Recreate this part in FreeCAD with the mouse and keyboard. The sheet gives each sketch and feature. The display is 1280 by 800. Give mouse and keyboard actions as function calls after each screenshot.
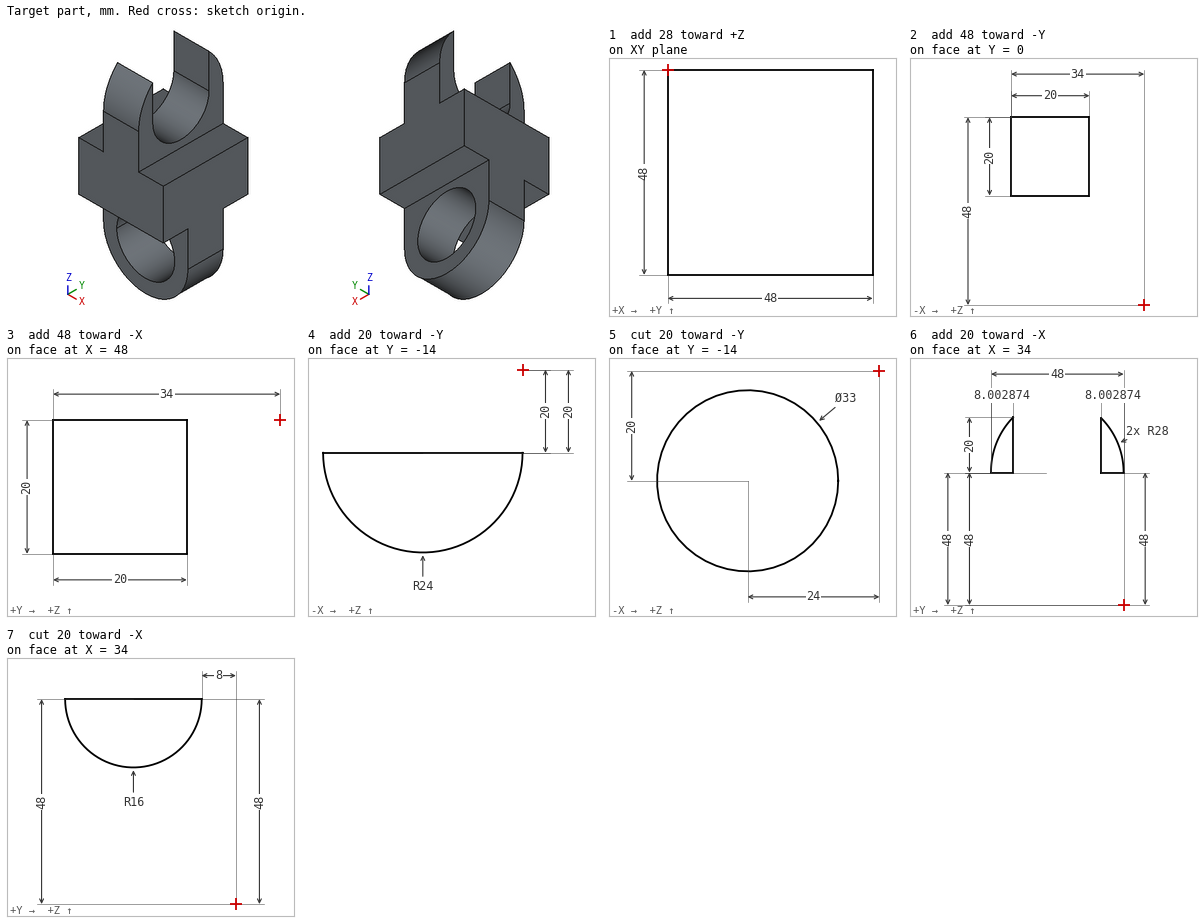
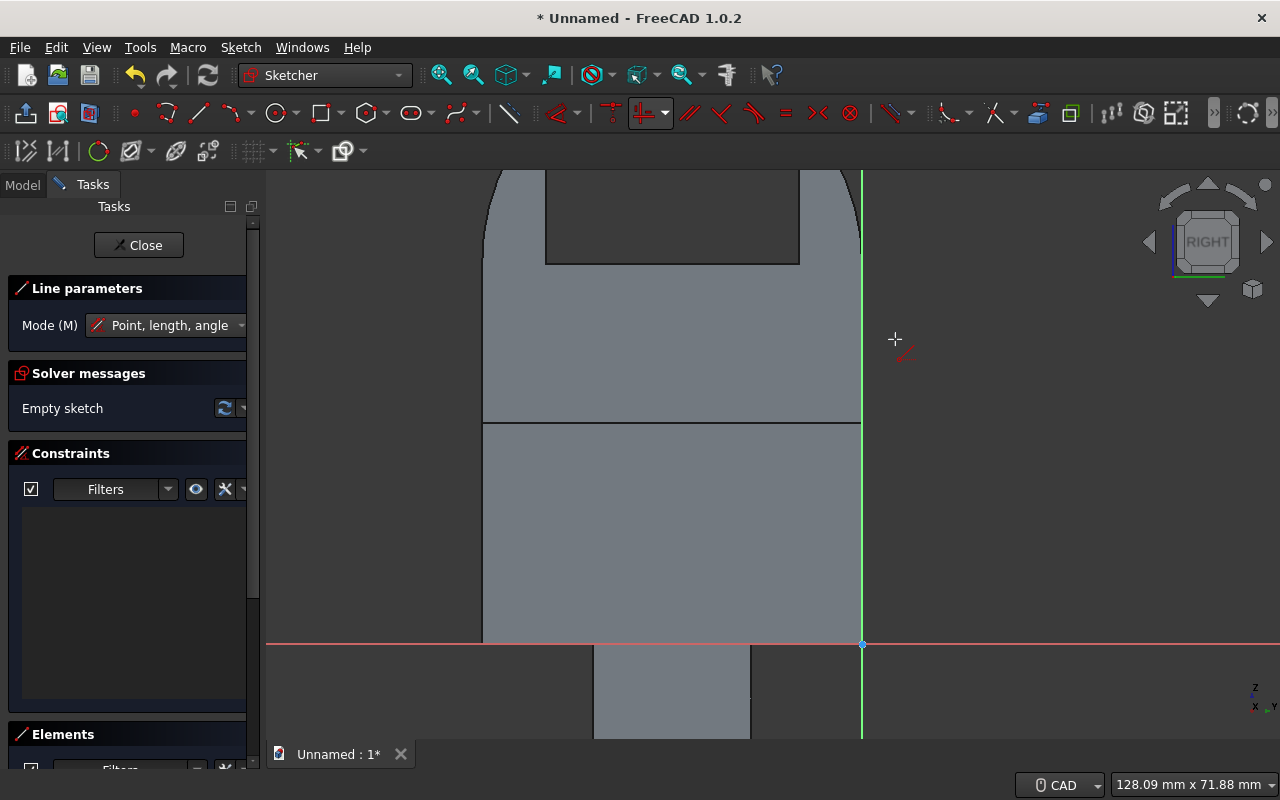
click(799, 264)
click(546, 264)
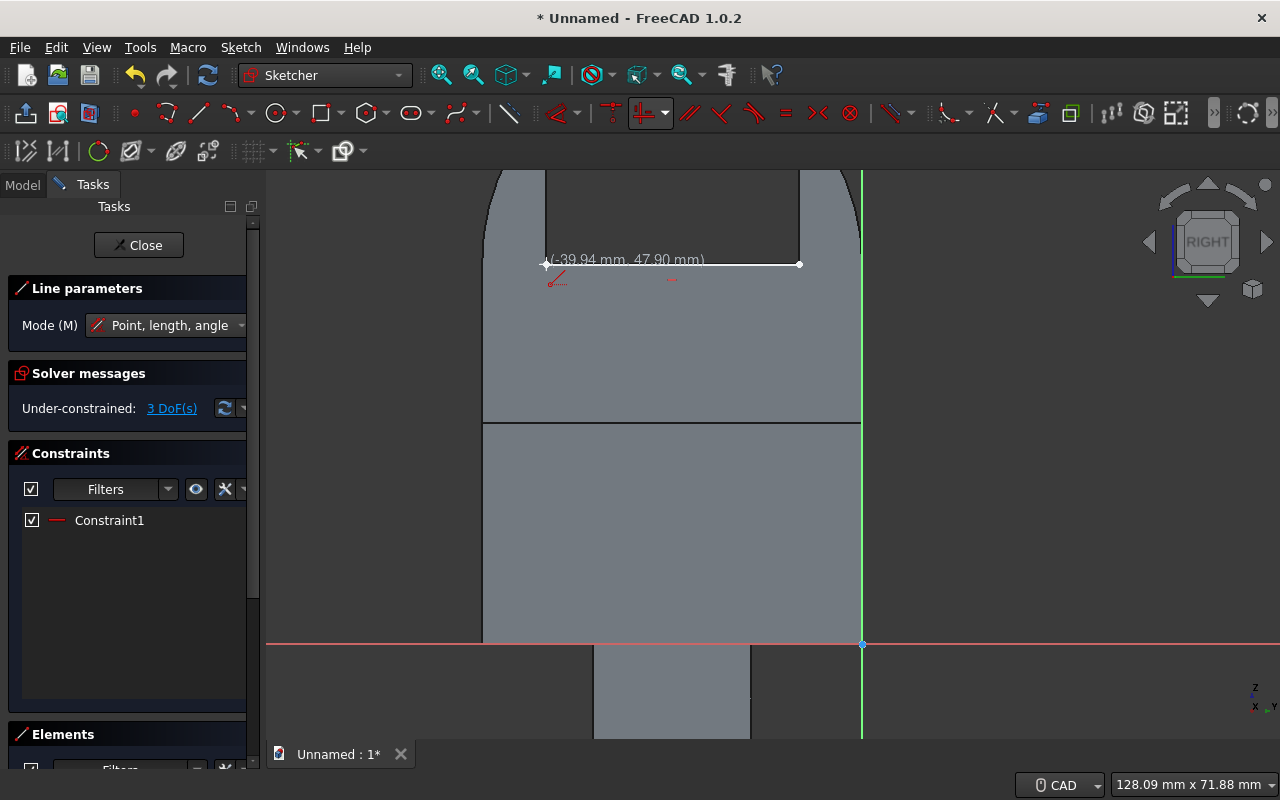
key(g)
key(3)
key(a)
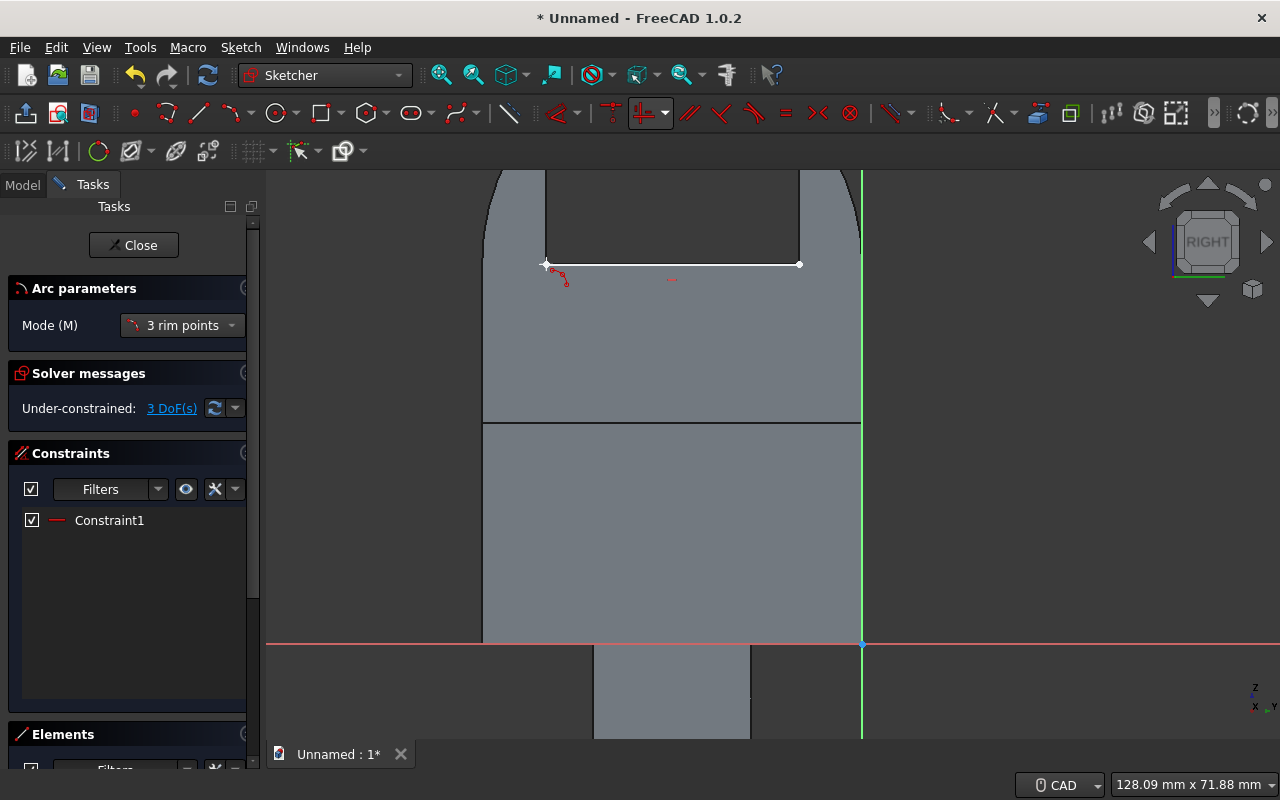
click(546, 265)
click(799, 265)
click(672, 391)
key(Escape)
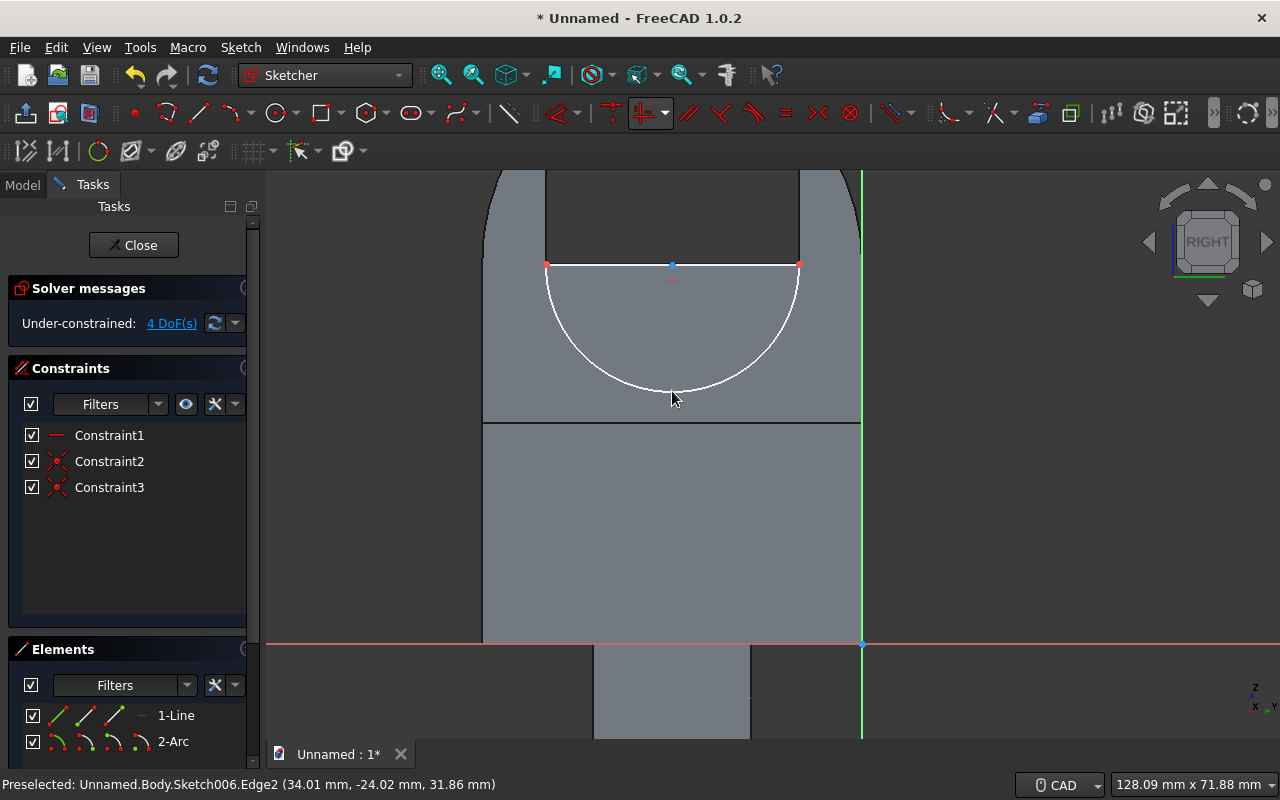
key(d)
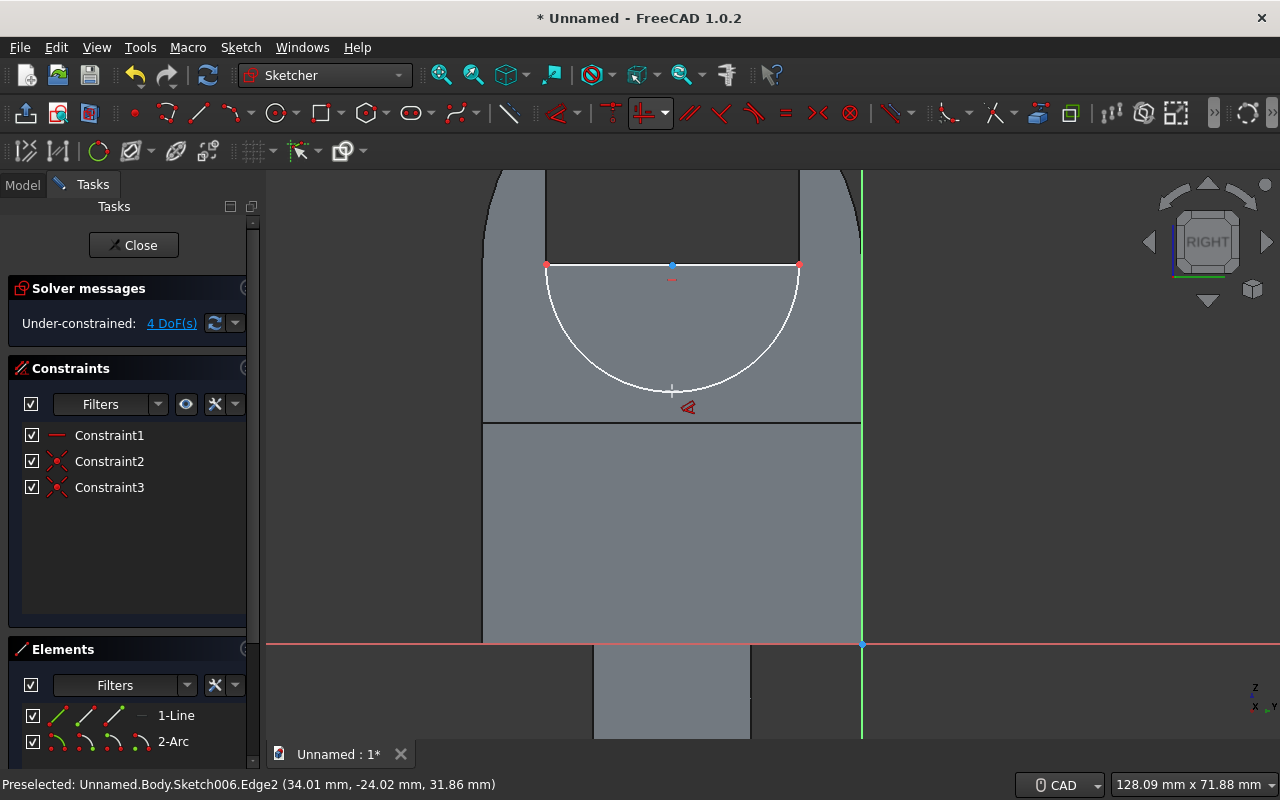
click(598, 368)
click(579, 394)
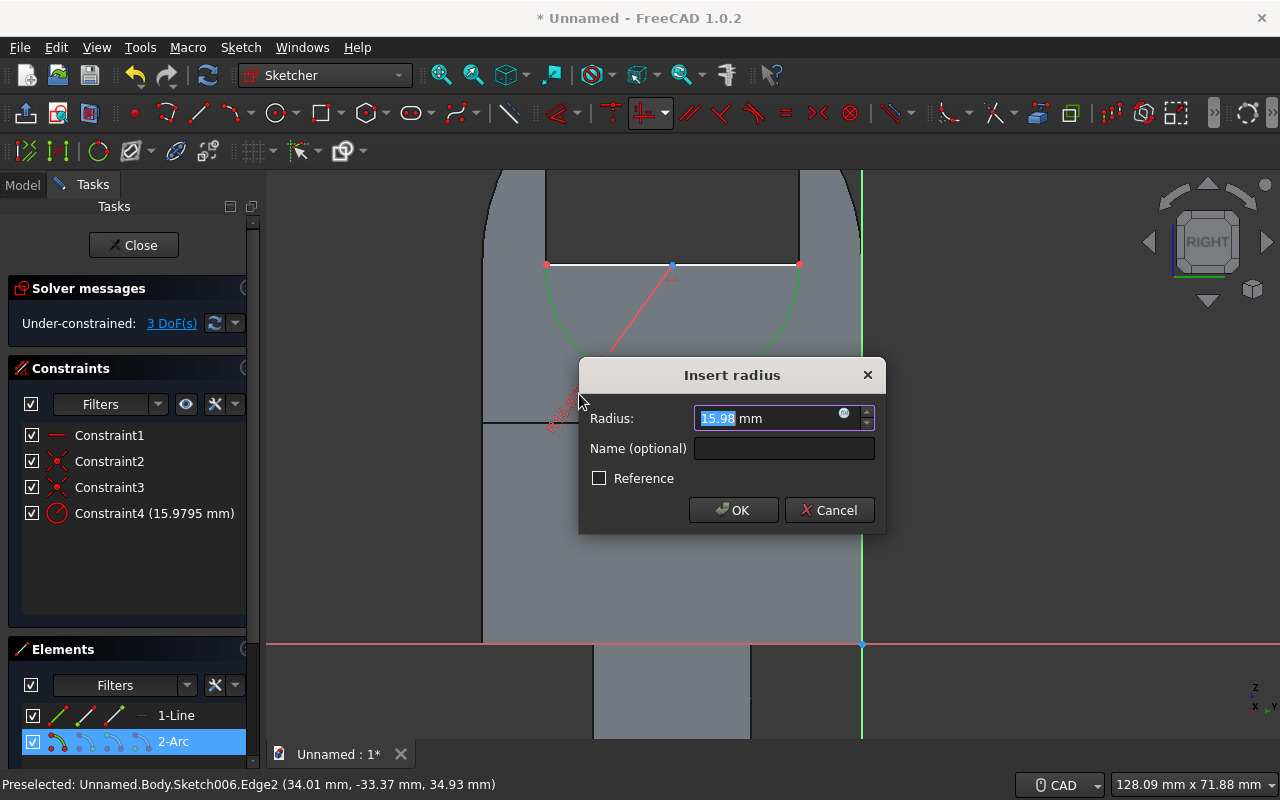
text(16)
key(Return)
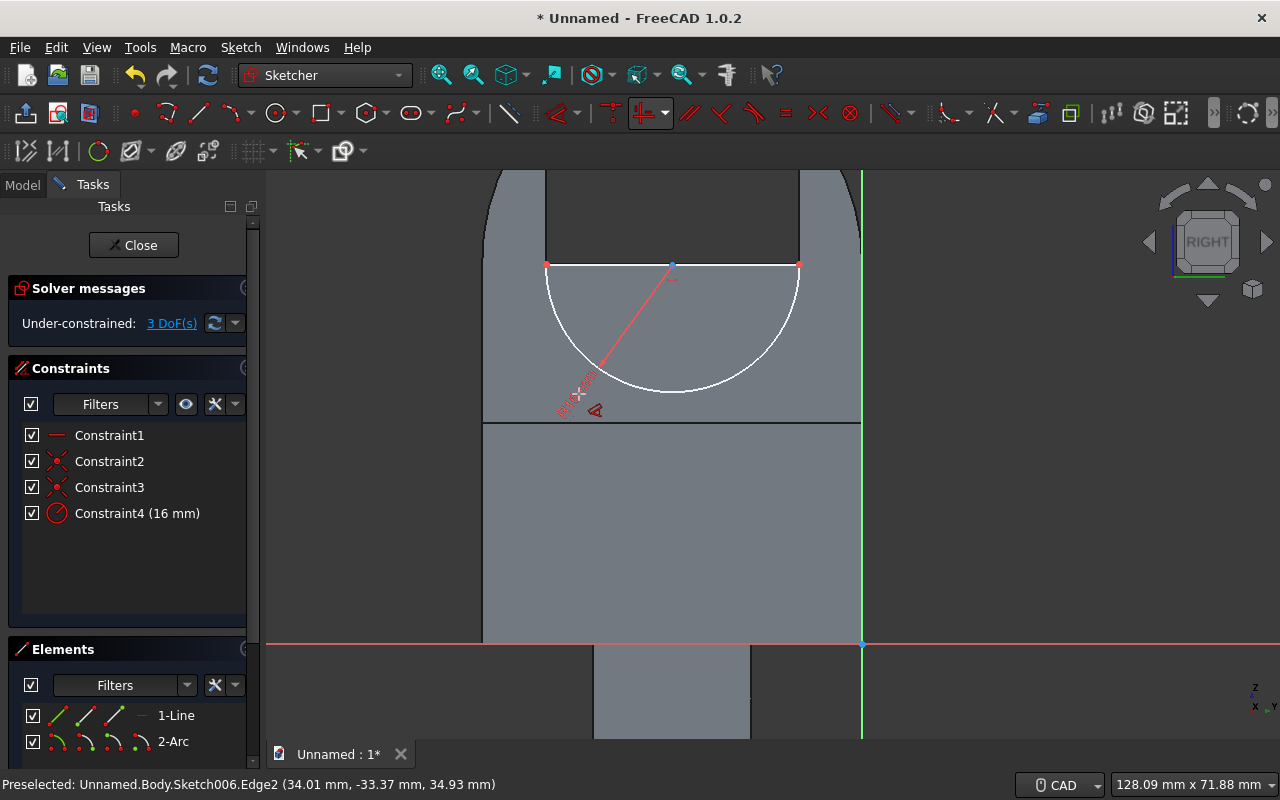
click(799, 265)
click(831, 678)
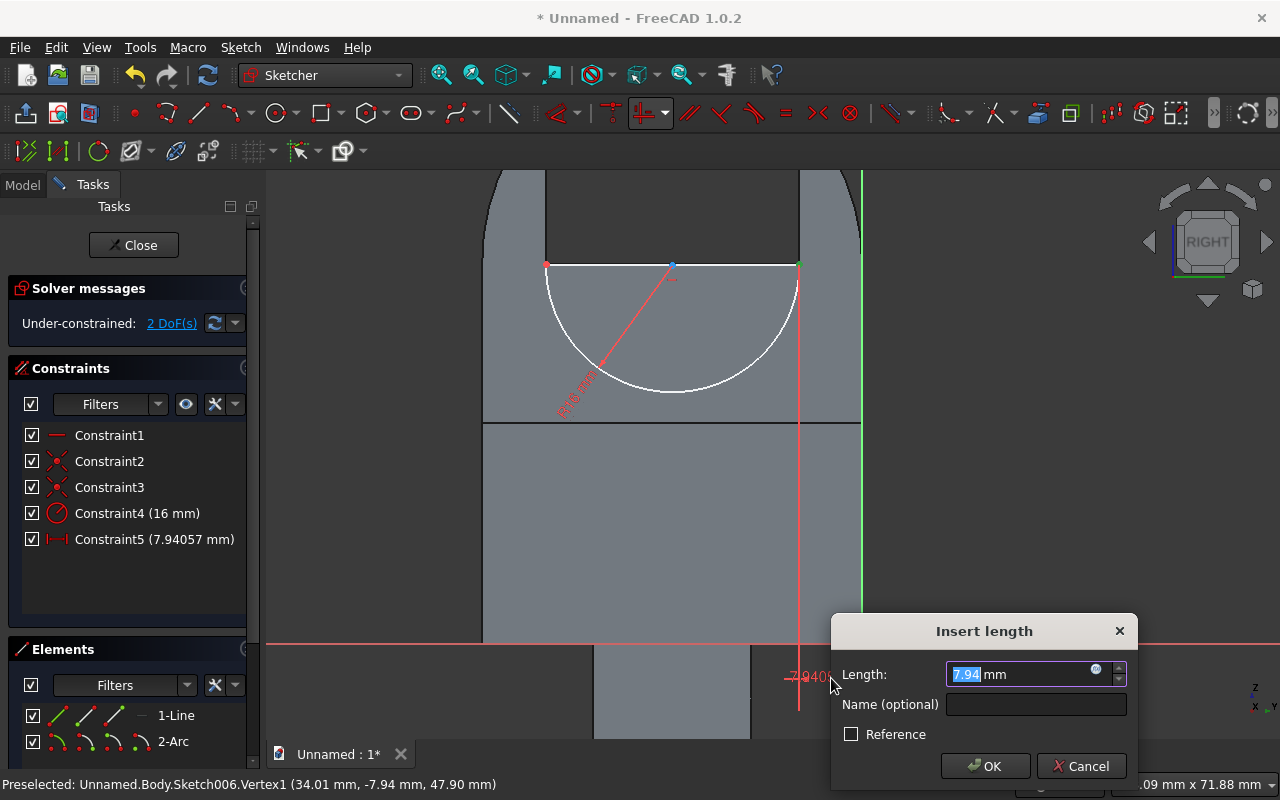
text(8)
key(Return)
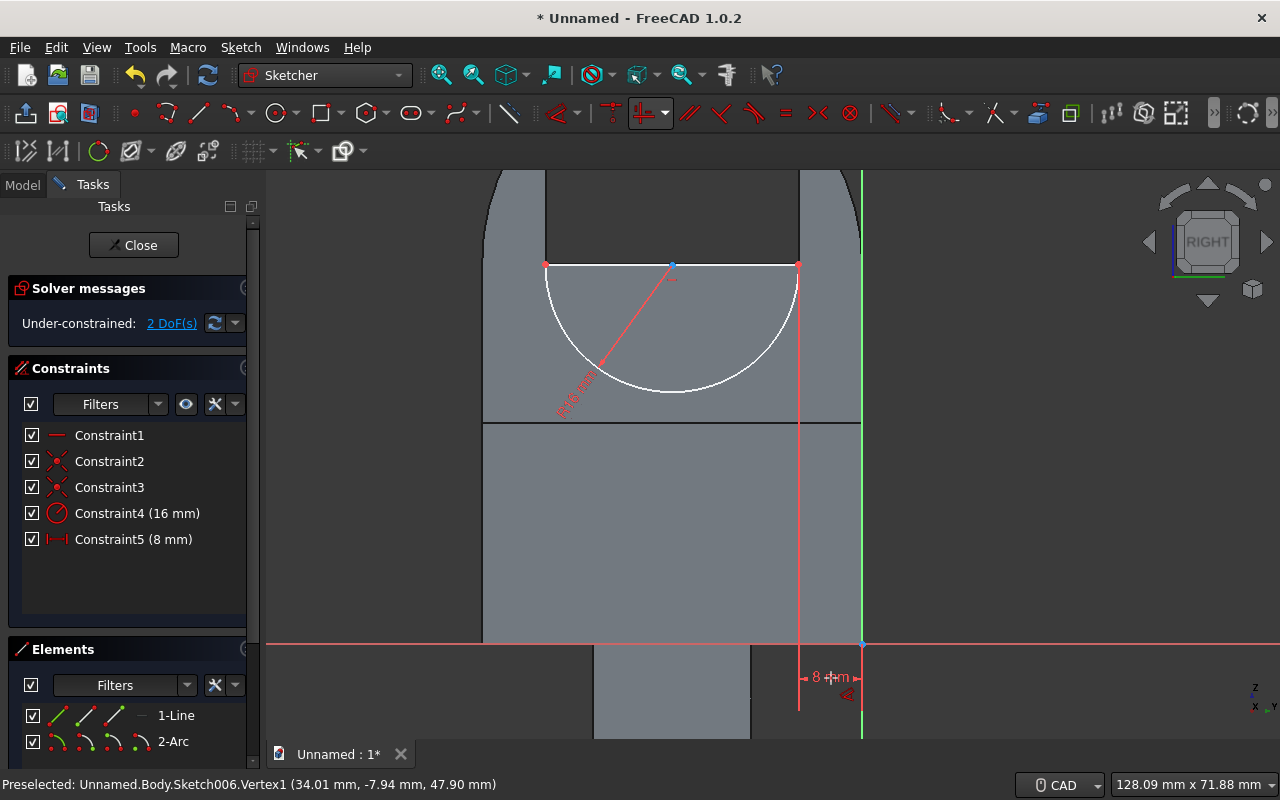
click(799, 265)
click(896, 455)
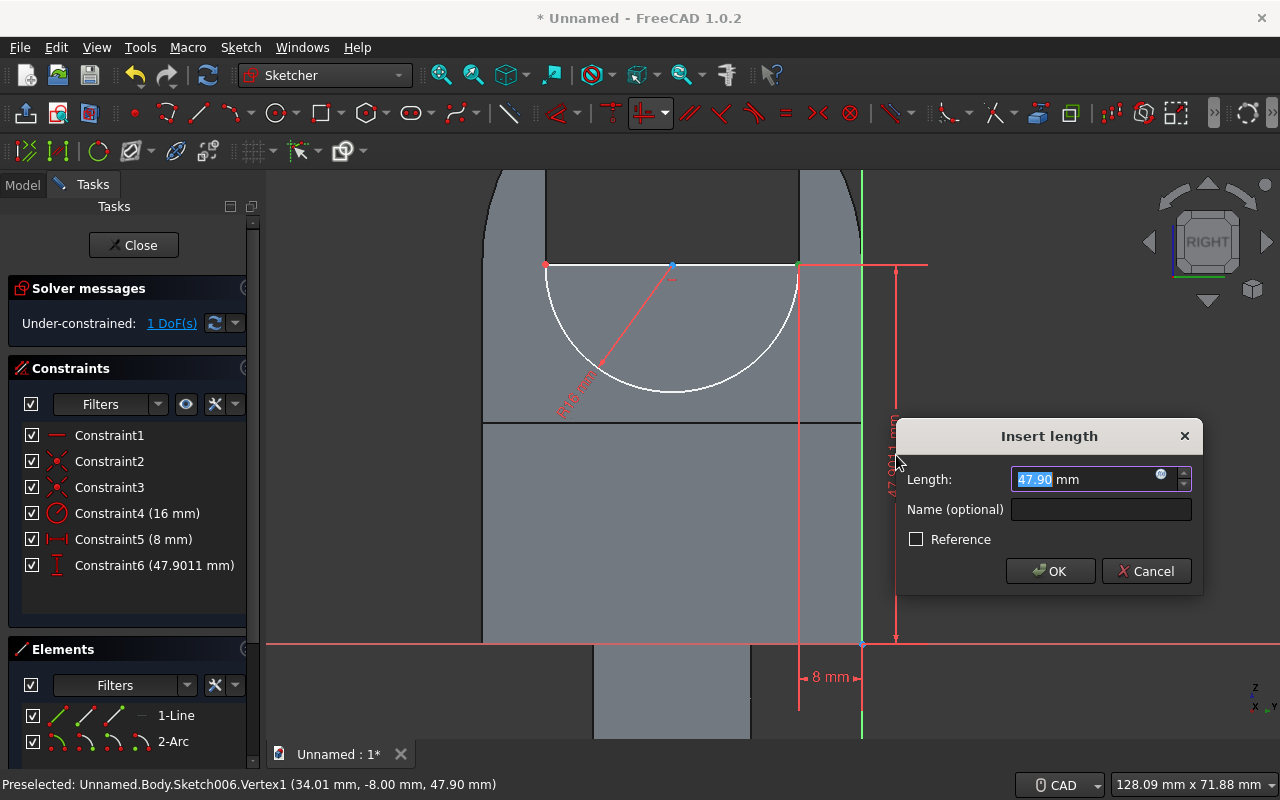
text(48)
key(Return)